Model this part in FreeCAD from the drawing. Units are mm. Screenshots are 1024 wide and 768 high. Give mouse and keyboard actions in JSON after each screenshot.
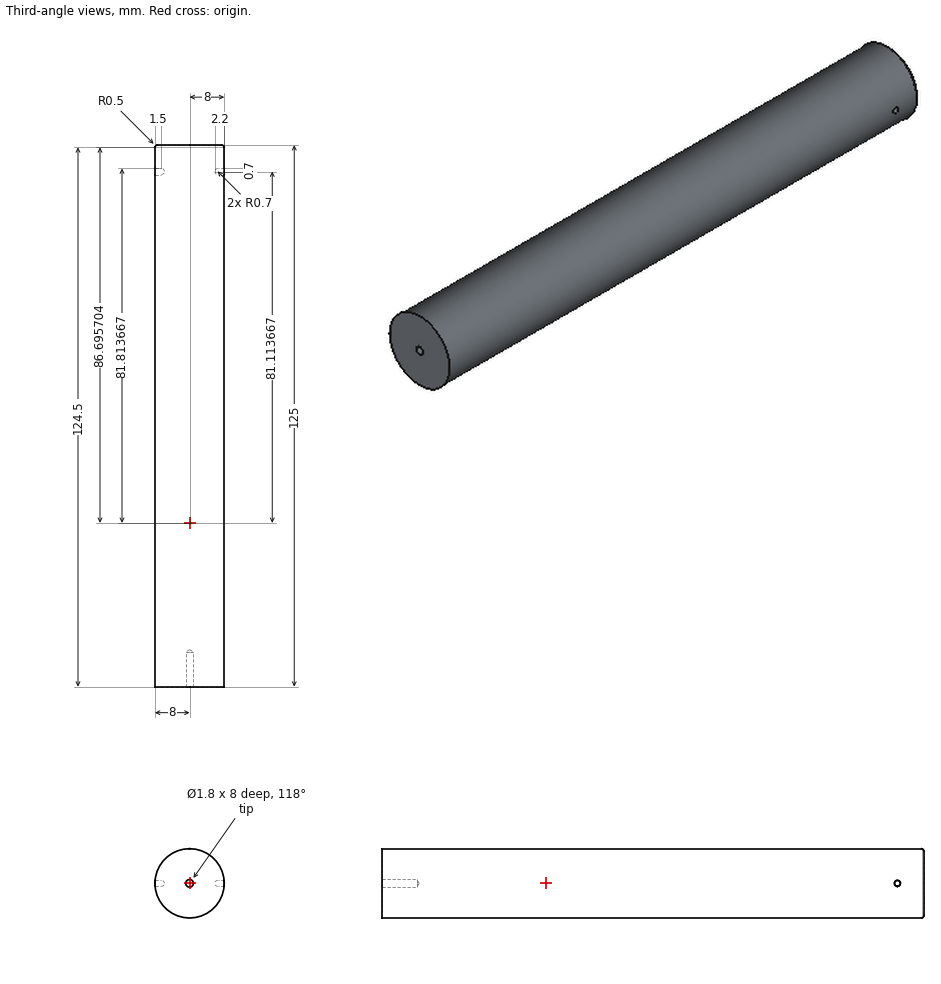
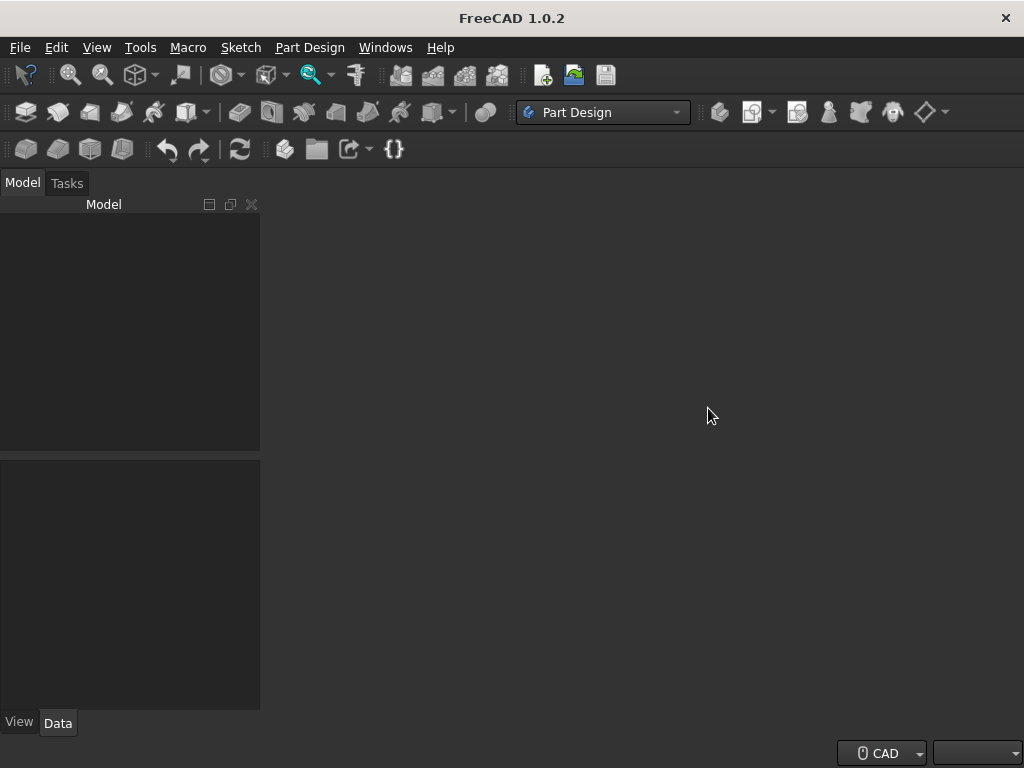
{"action": "left_click", "coordinate": [542, 76]}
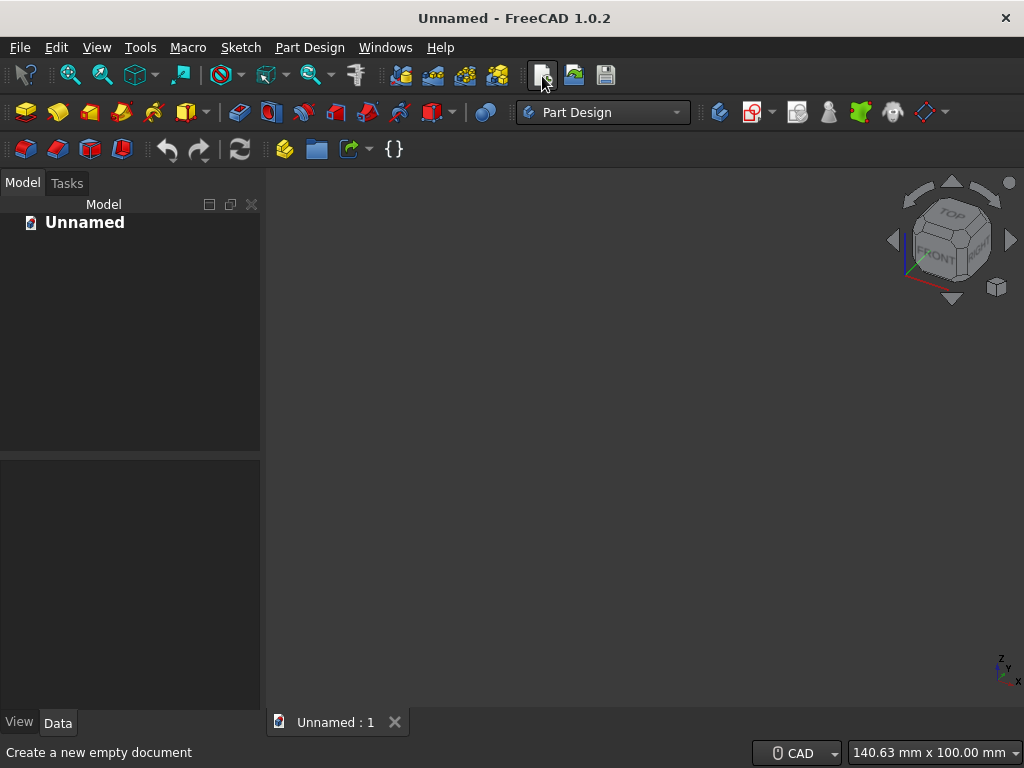
{"action": "left_click", "coordinate": [752, 112]}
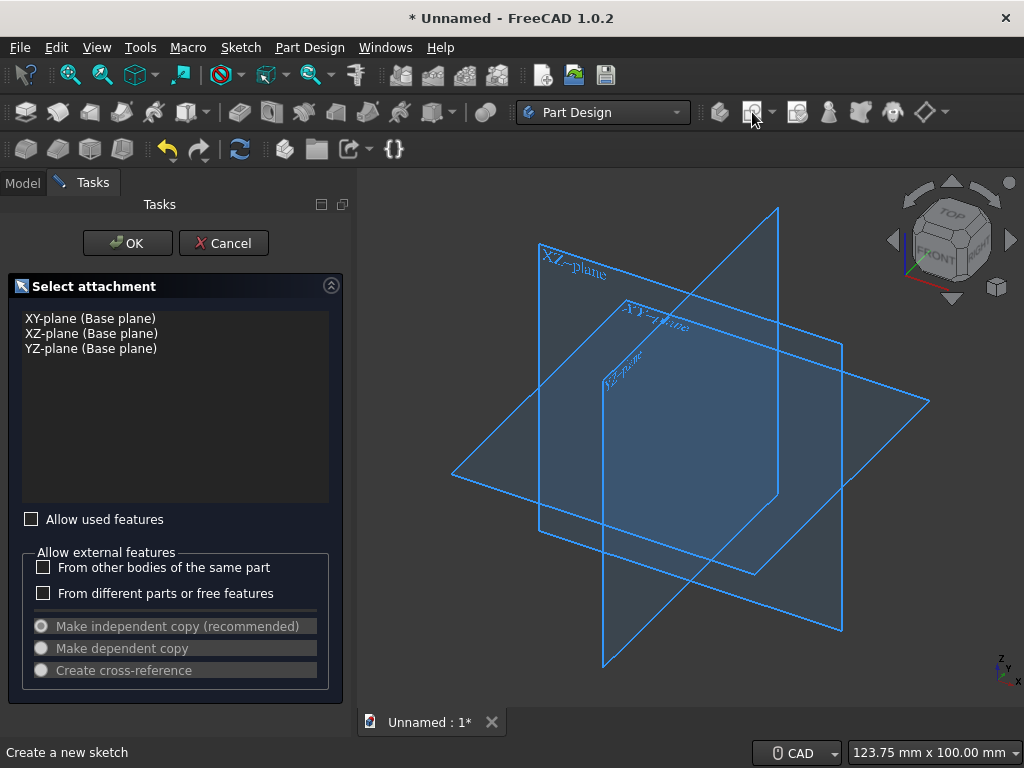
{"action": "left_click", "coordinate": [82, 318]}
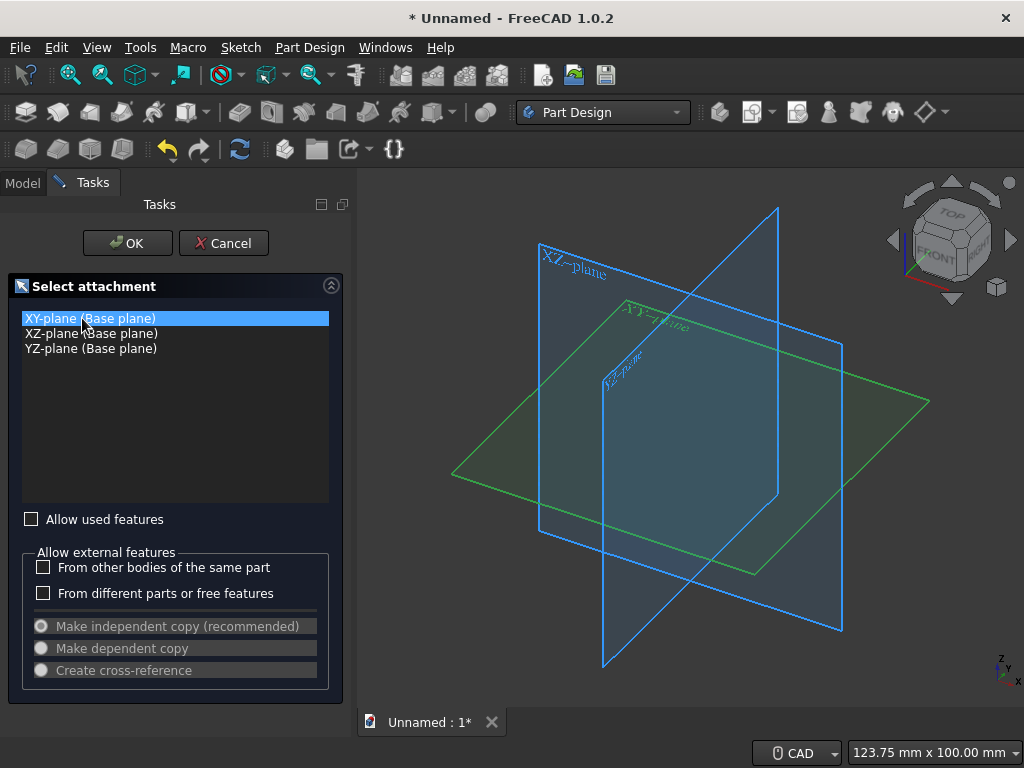
{"action": "left_click", "coordinate": [128, 243]}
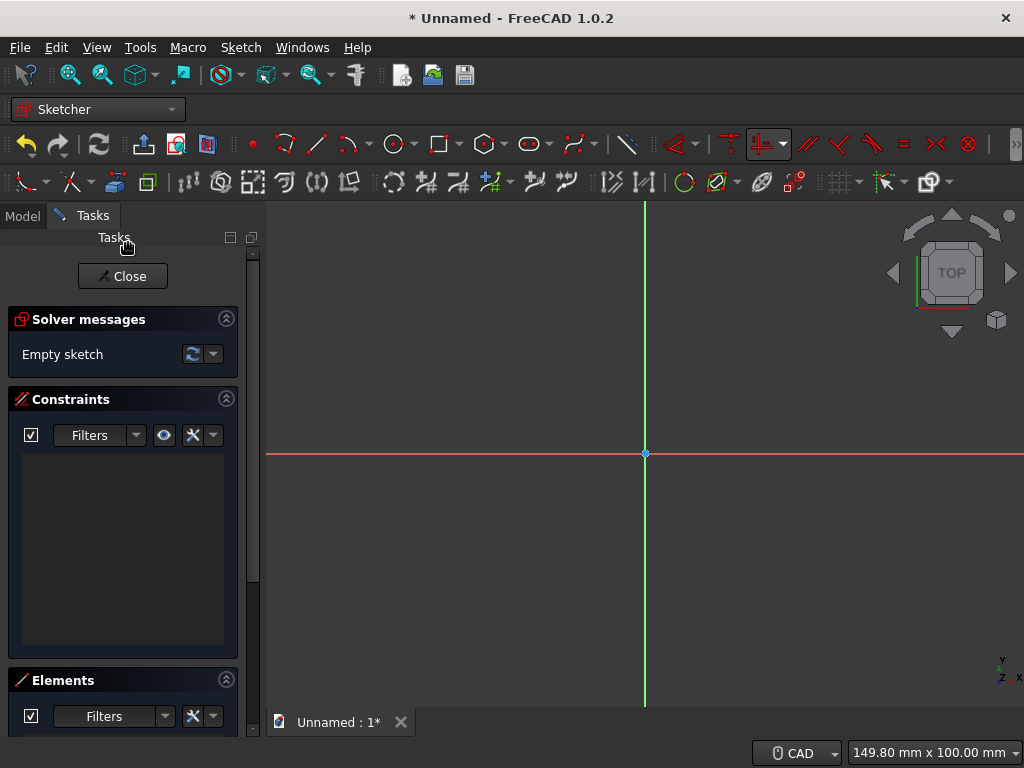
{"action": "scroll", "coordinate": [518, 606], "scroll_direction": "down", "scroll_amount": 3}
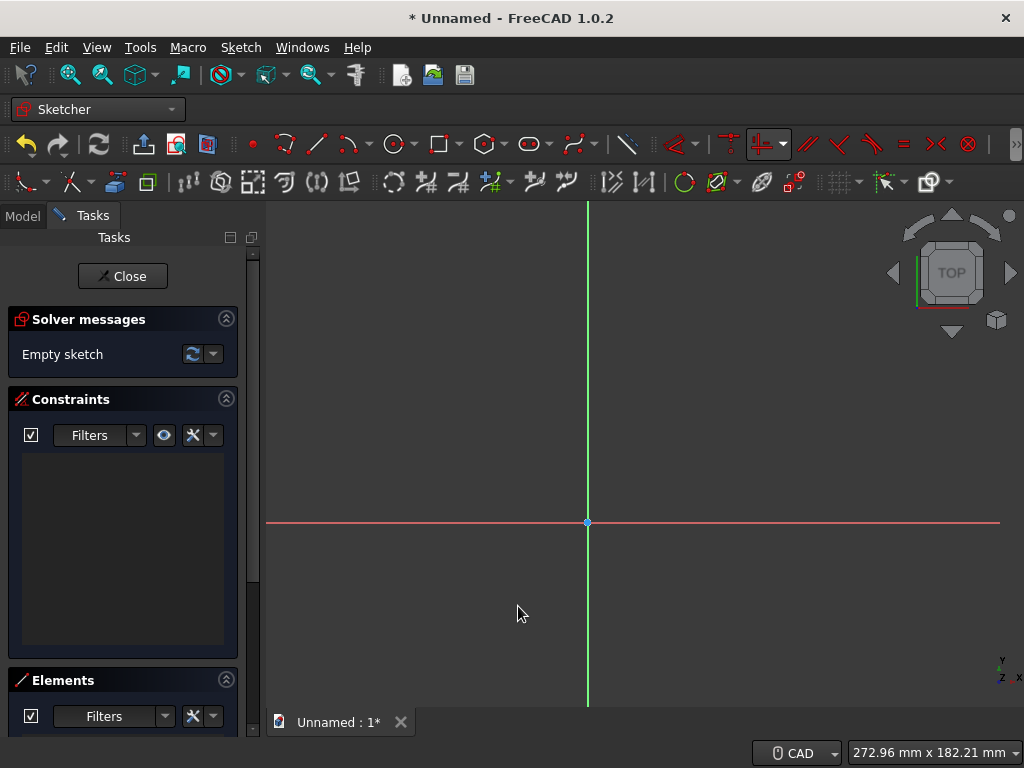
{"action": "left_click", "coordinate": [286, 144]}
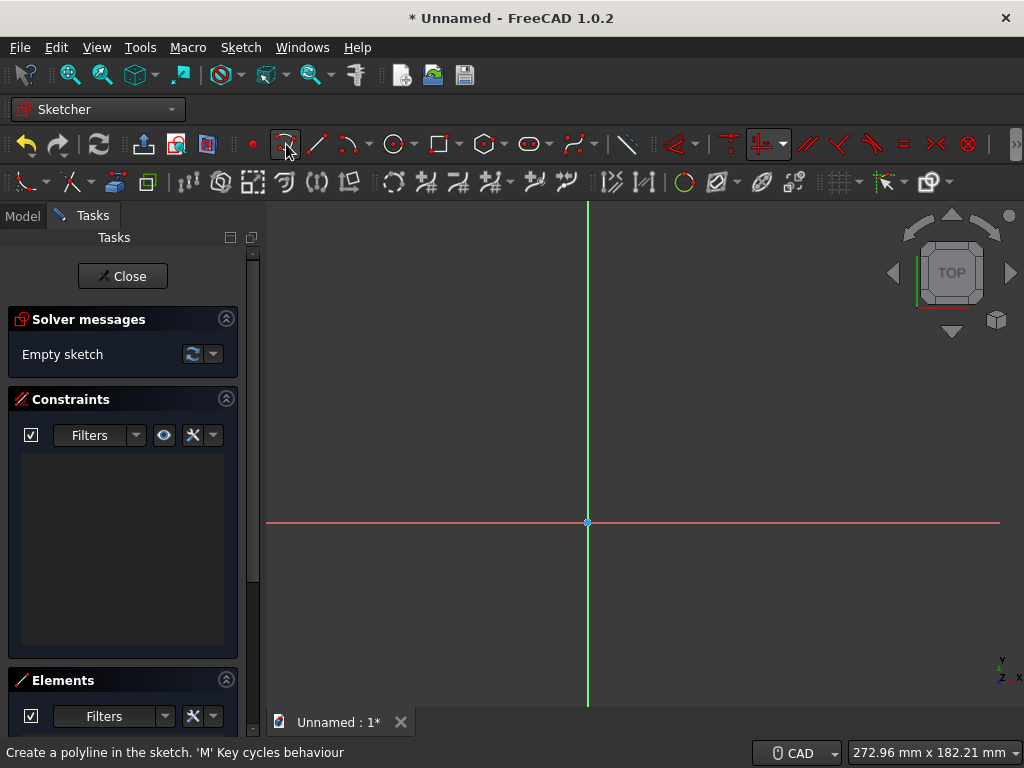
{"action": "left_click", "coordinate": [566, 282]}
{"action": "left_click", "coordinate": [566, 628]}
{"action": "left_click", "coordinate": [588, 628]}
{"action": "left_click", "coordinate": [579, 281]}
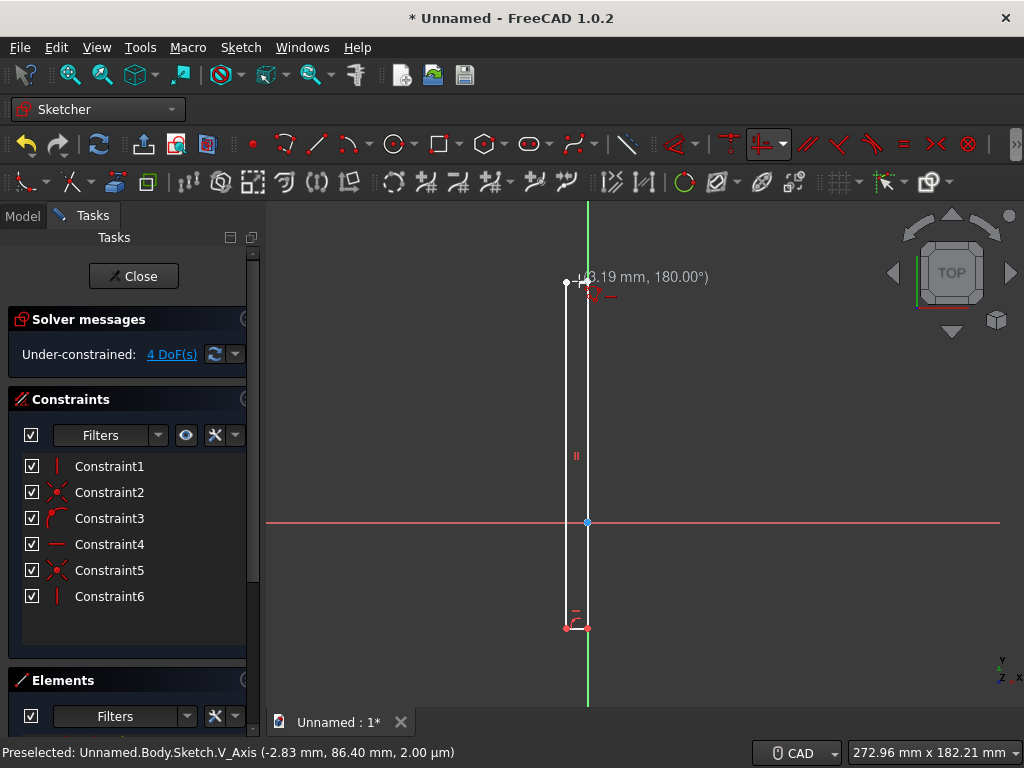
{"action": "scroll", "coordinate": [567, 281], "scroll_direction": "up", "scroll_amount": 11}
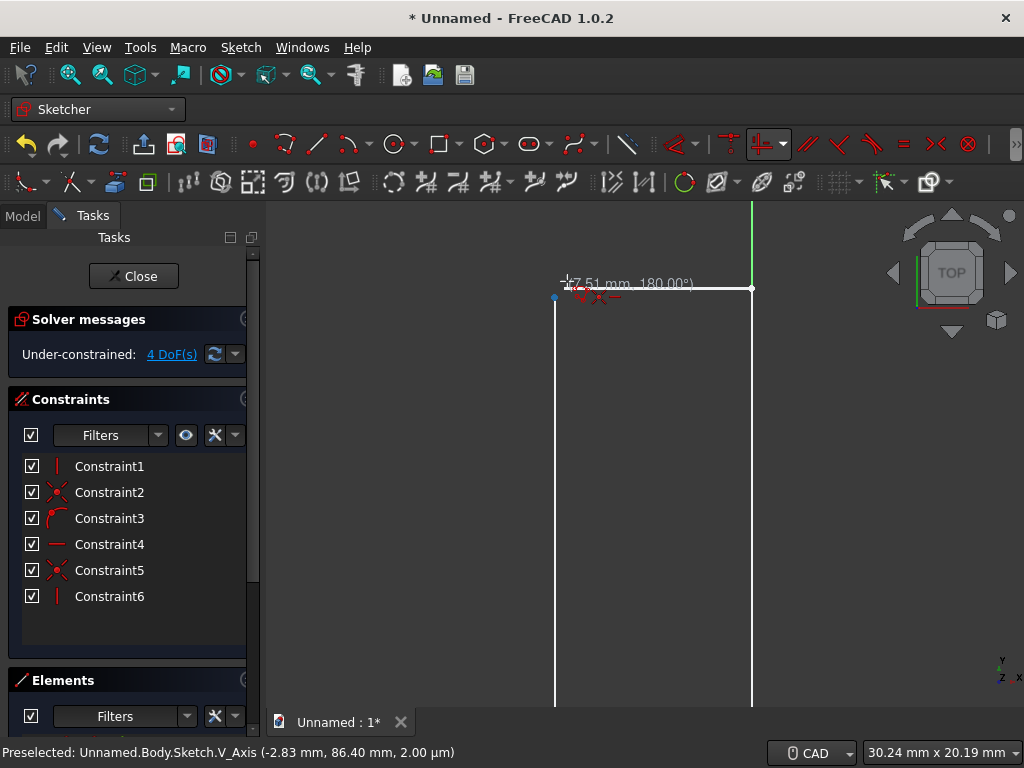
{"action": "left_click", "coordinate": [564, 280]}
{"action": "right_click", "coordinate": [564, 280]}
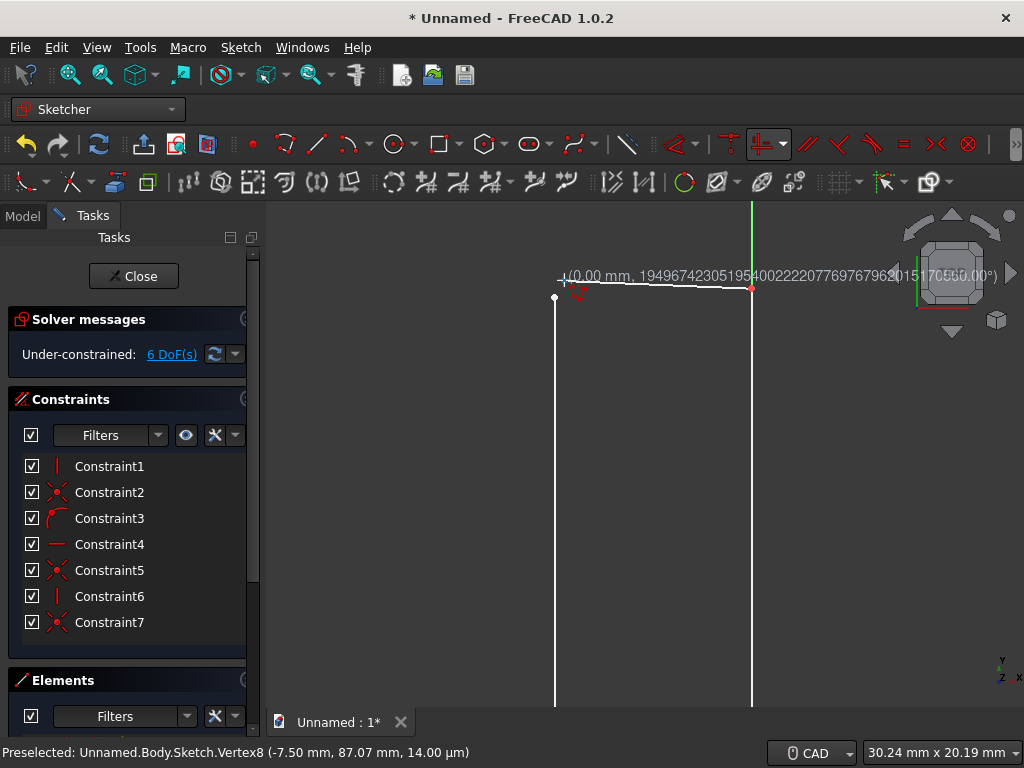
{"action": "key", "text": "g 3 a"}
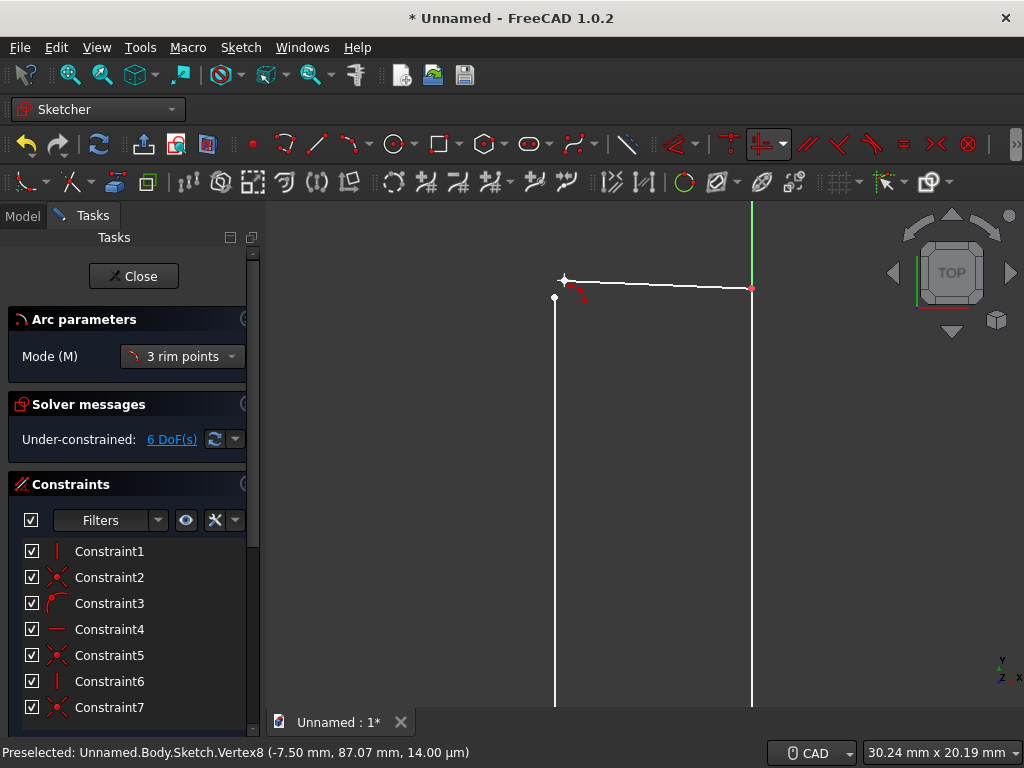
{"action": "left_click", "coordinate": [564, 281]}
{"action": "left_click", "coordinate": [555, 289]}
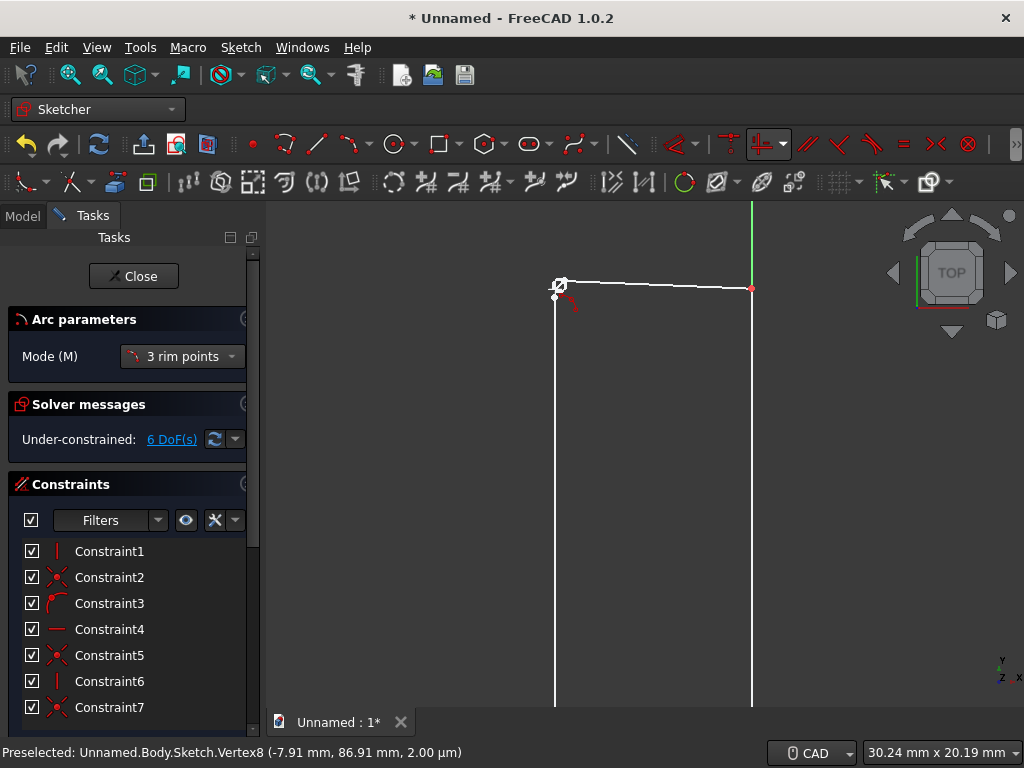
{"action": "scroll", "coordinate": [555, 282], "scroll_direction": "up", "scroll_amount": 8}